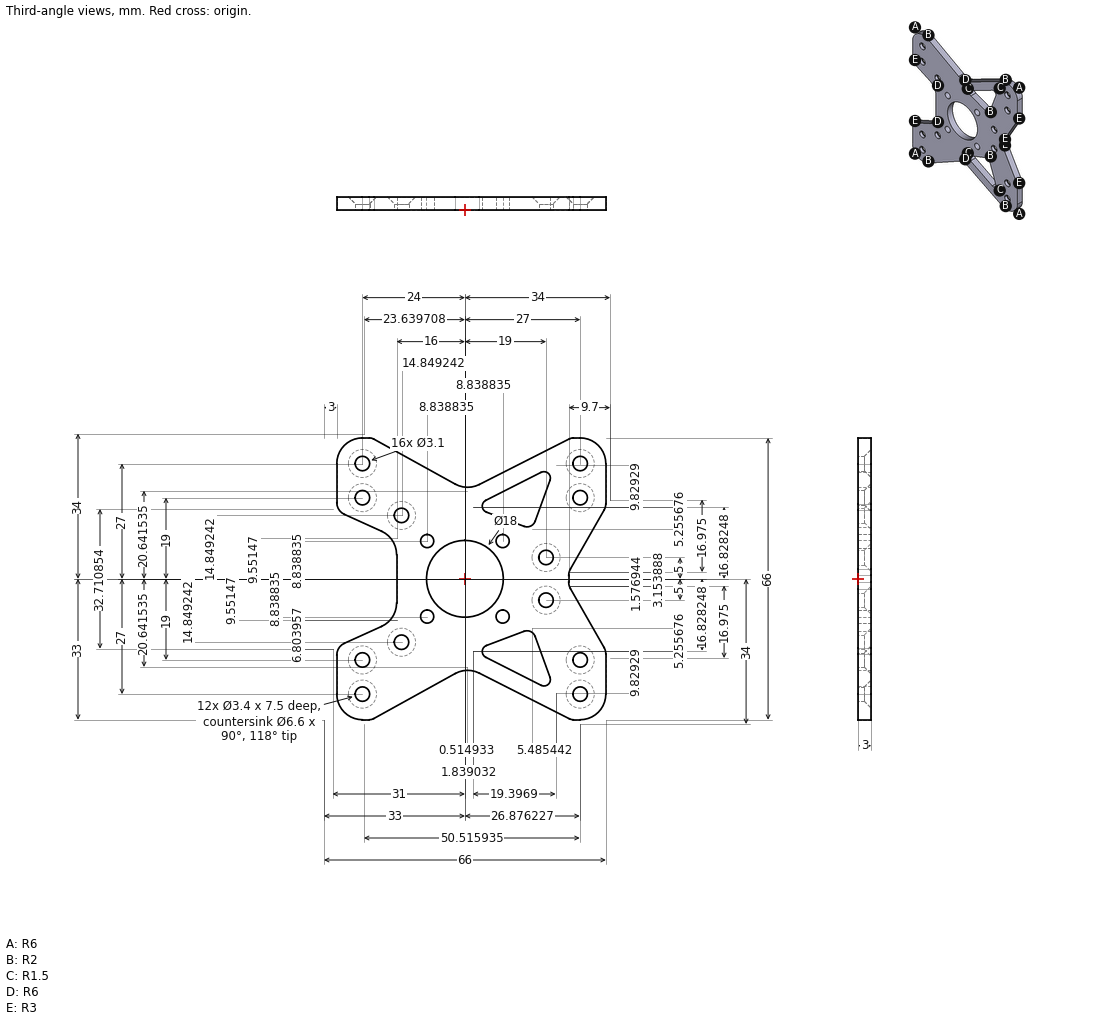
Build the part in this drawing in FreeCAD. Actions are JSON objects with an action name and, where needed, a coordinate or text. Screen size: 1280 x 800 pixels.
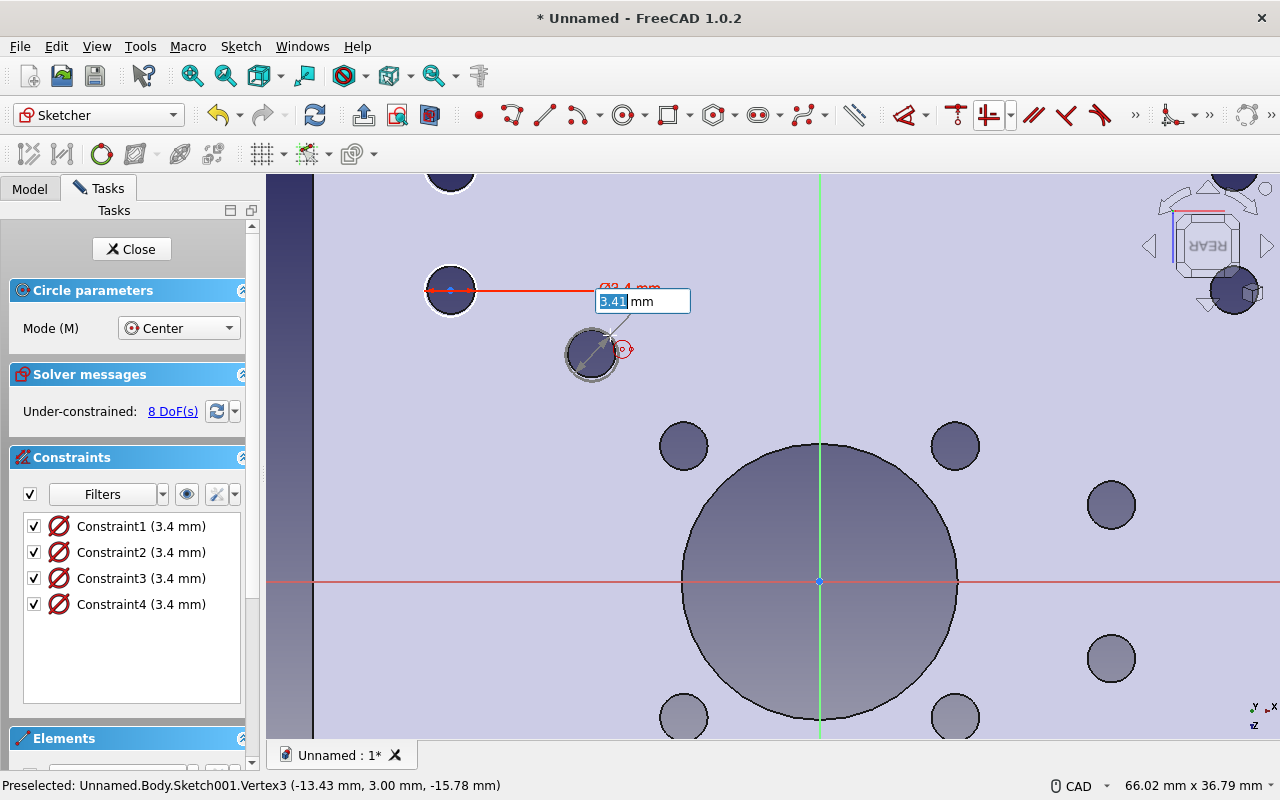
{"action": "type", "text": "3.4"}
{"action": "key", "text": "Return"}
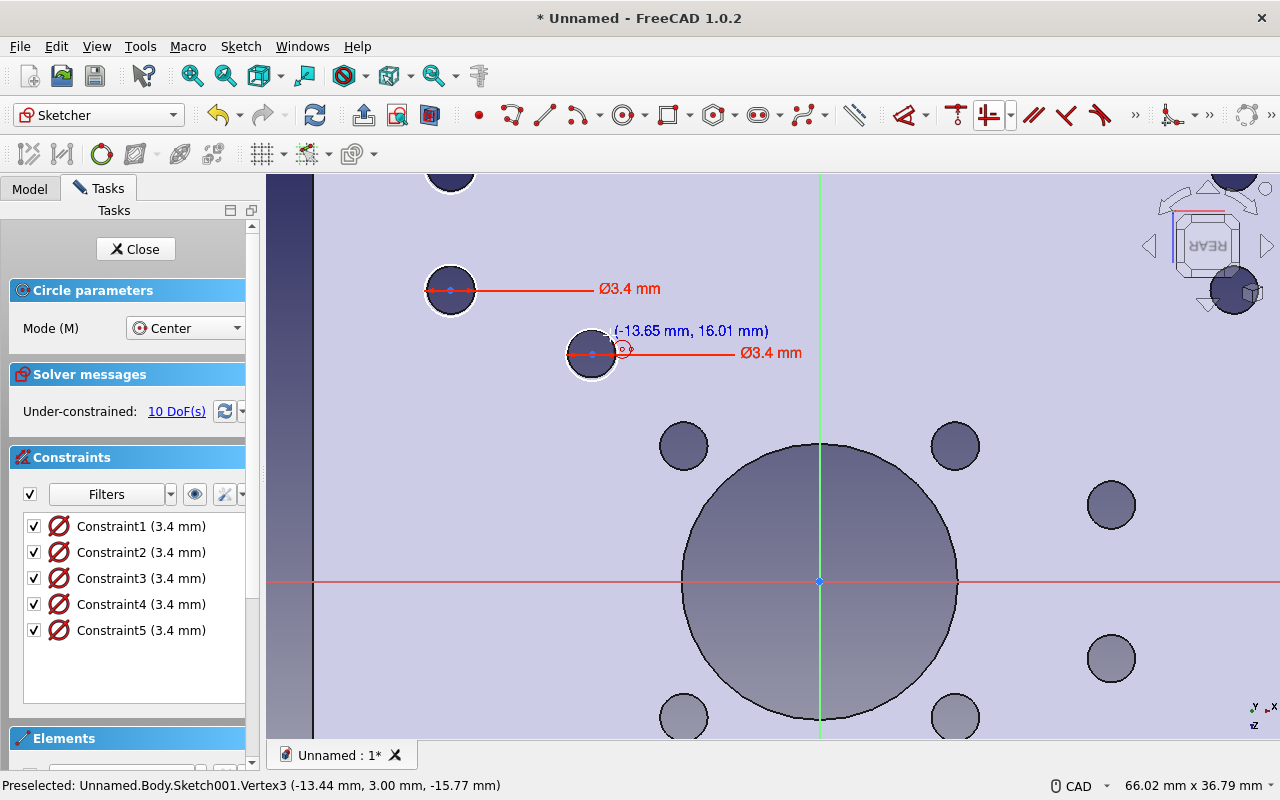
{"action": "scroll", "coordinate": [592, 354], "scroll_direction": "down", "scroll_amount": 4}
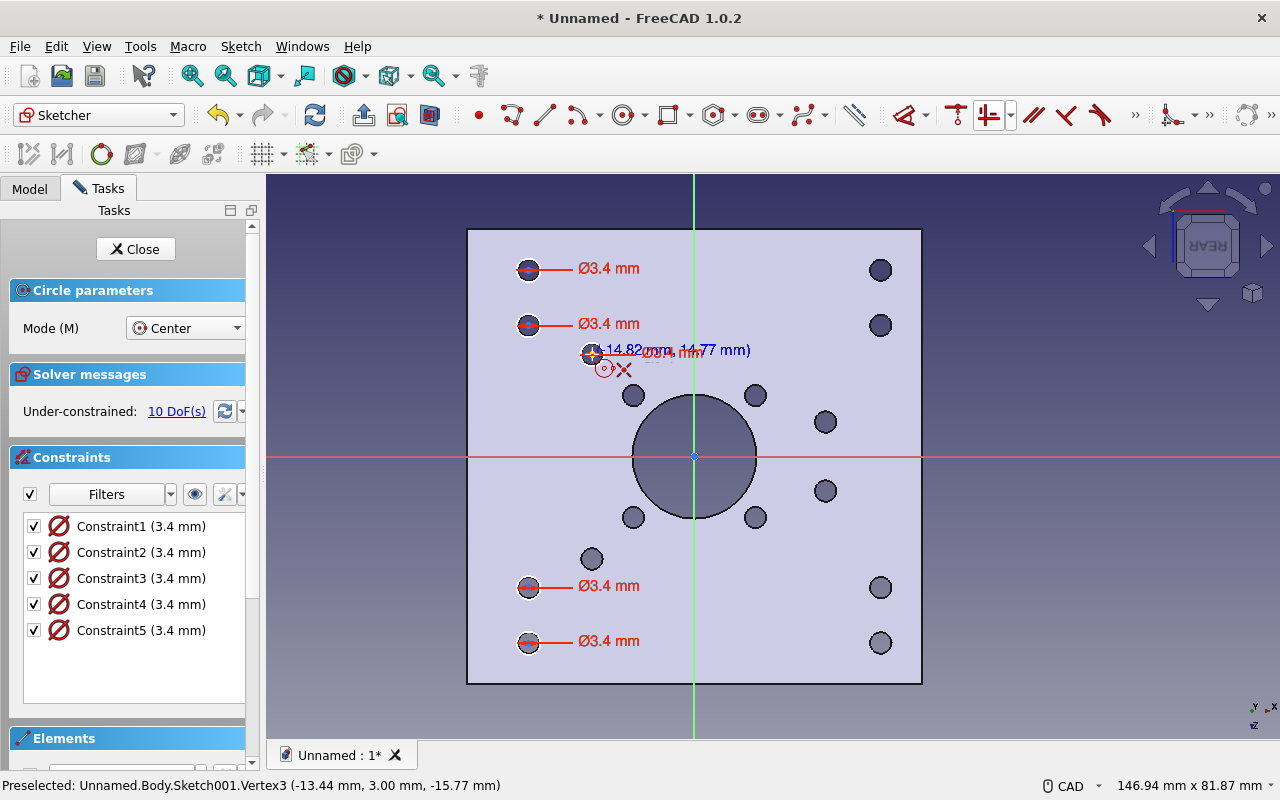
{"action": "scroll", "coordinate": [592, 559], "scroll_direction": "up", "scroll_amount": 4}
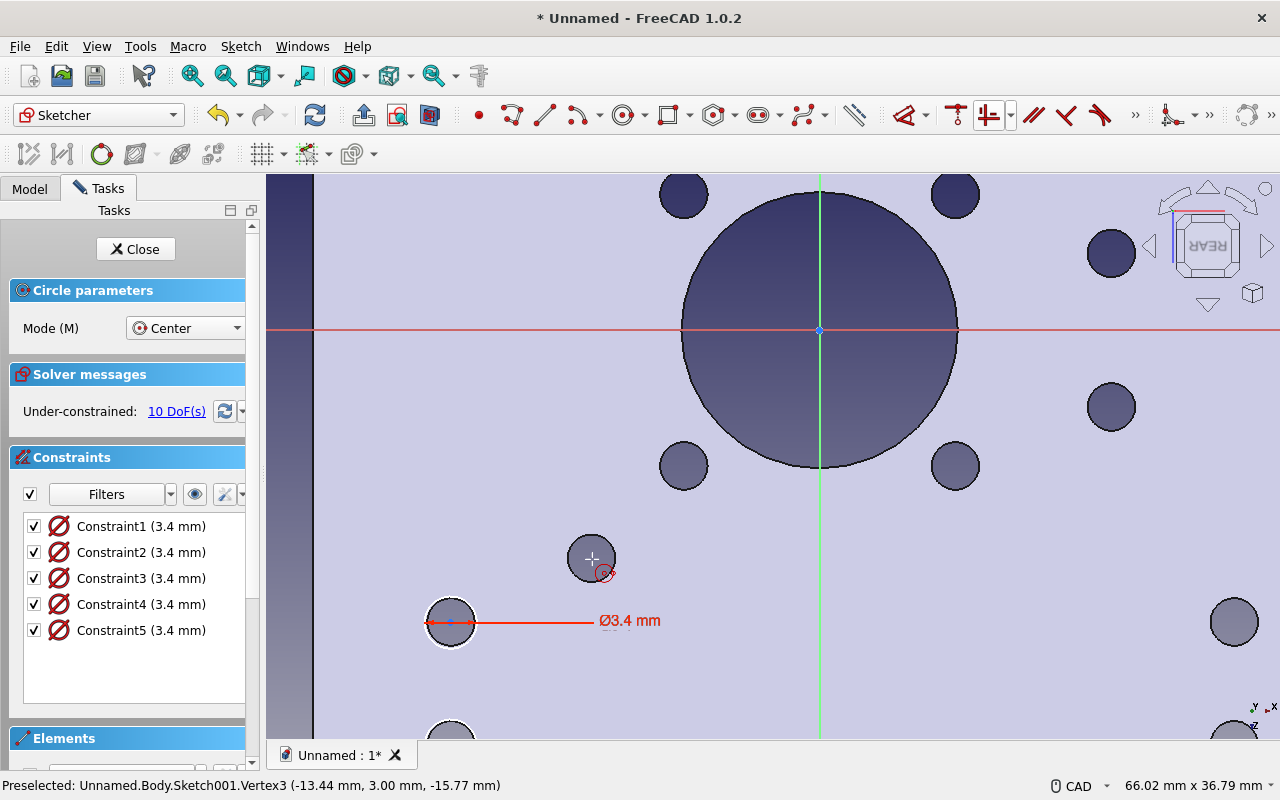
{"action": "left_click", "coordinate": [592, 558]}
{"action": "mouse_move", "coordinate": [610, 540]}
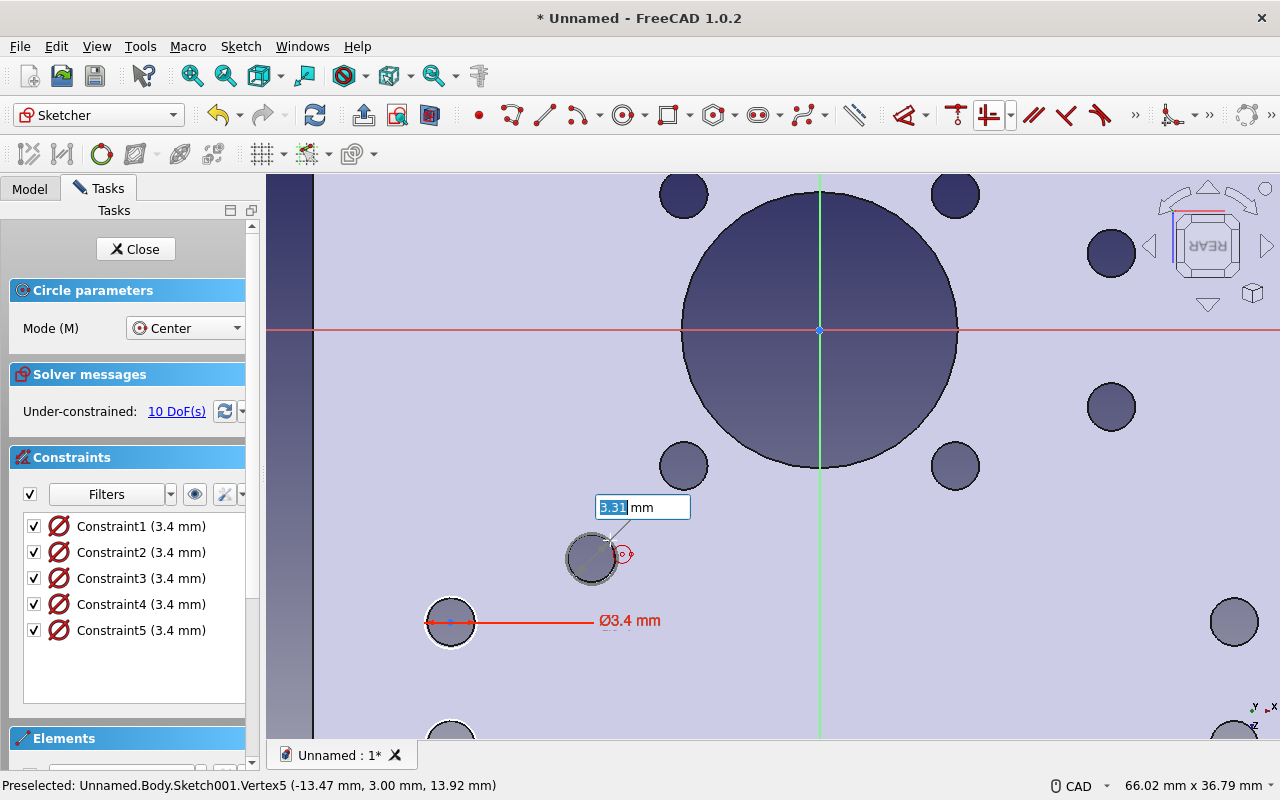
{"action": "type", "text": "3.4"}
{"action": "key", "text": "Return"}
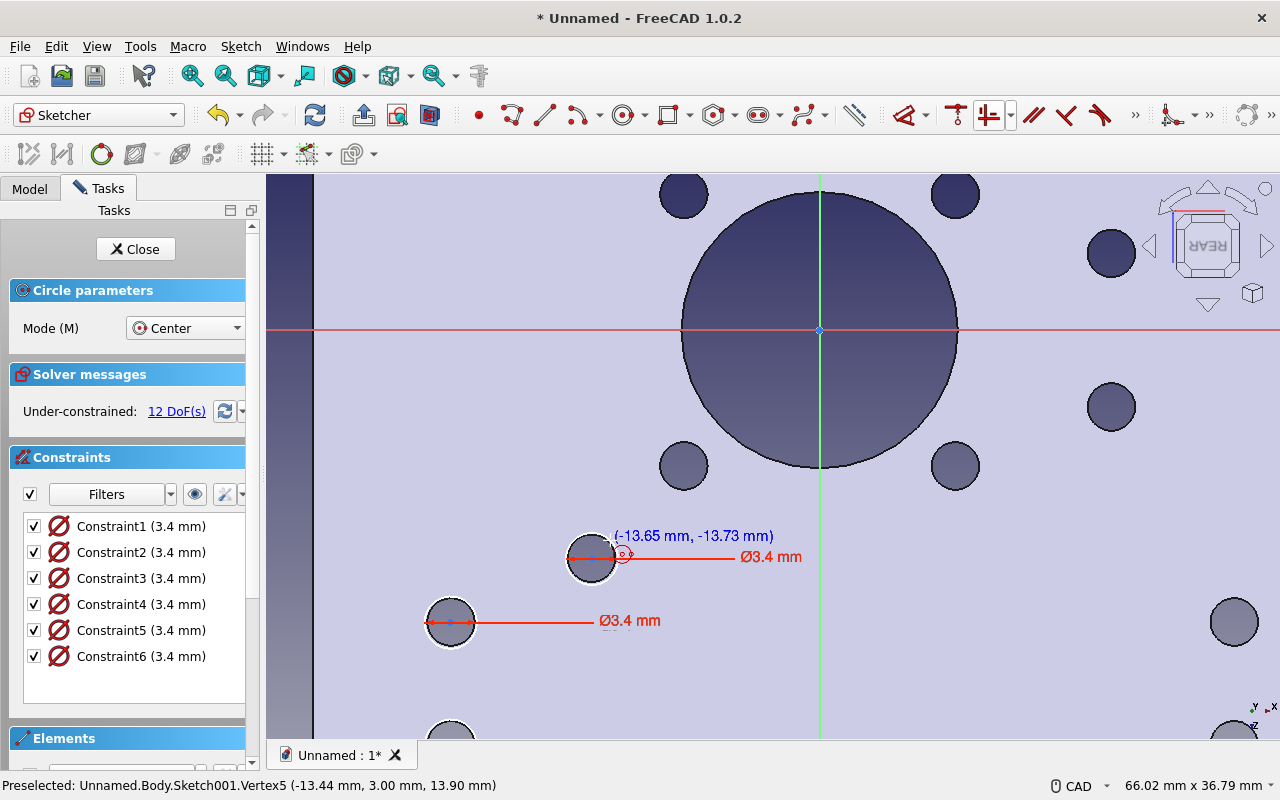
{"action": "left_click", "coordinate": [1111, 407]}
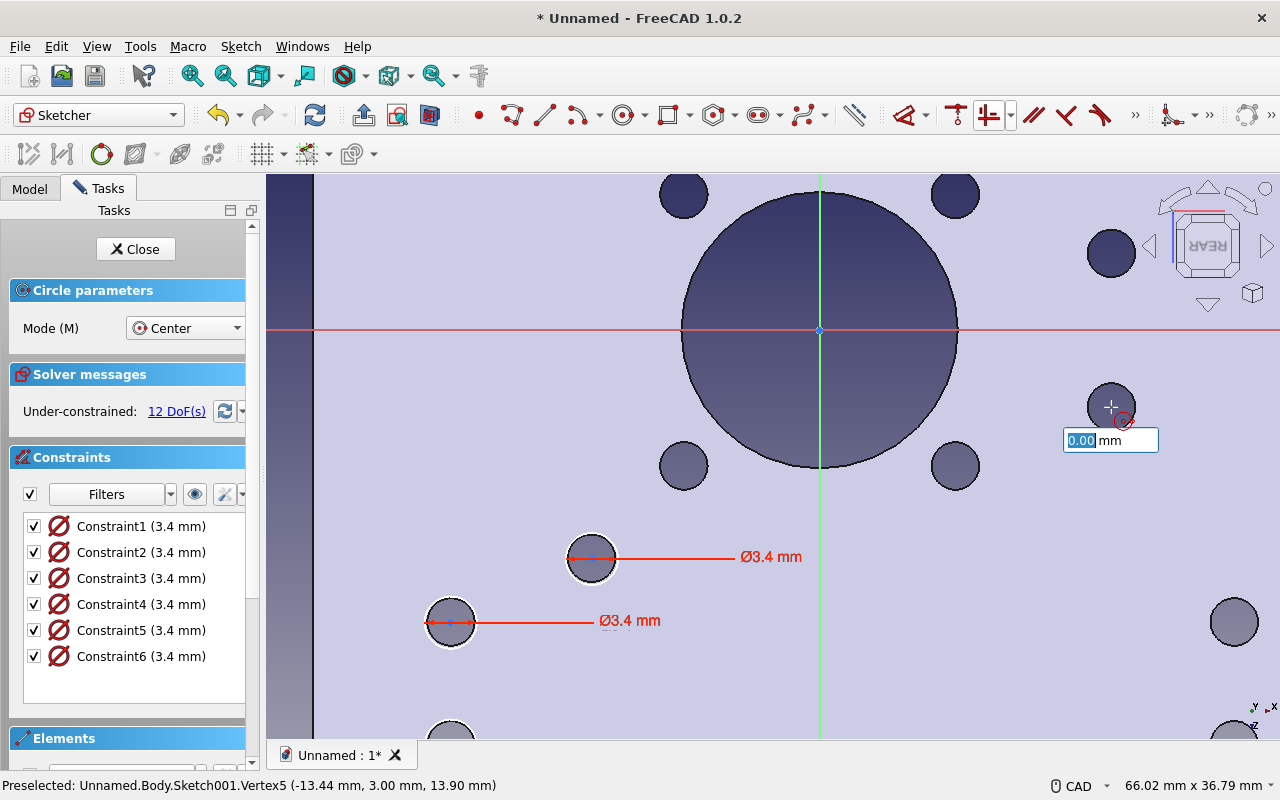
{"action": "scroll", "coordinate": [592, 560], "scroll_direction": "down", "scroll_amount": 4}
{"action": "mouse_move", "coordinate": [834, 483]}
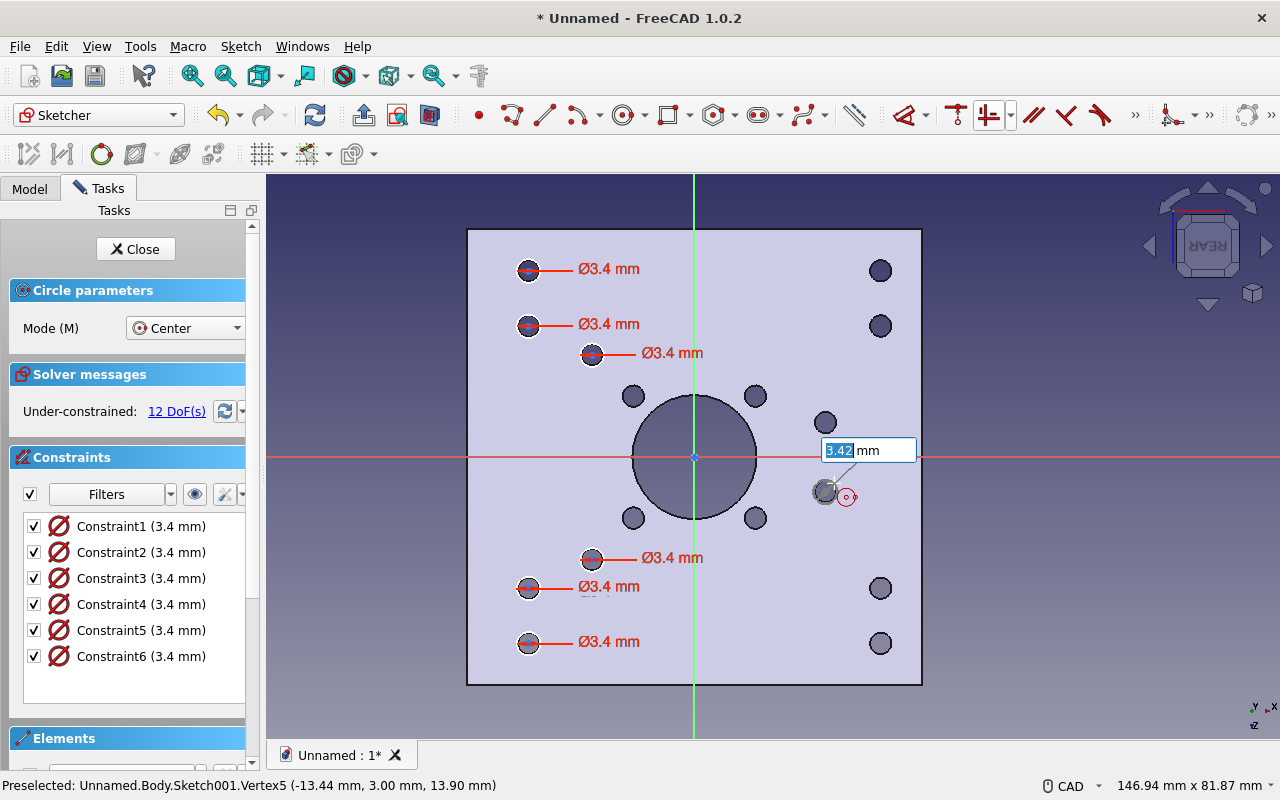
{"action": "type", "text": "3.4"}
{"action": "key", "text": "Return"}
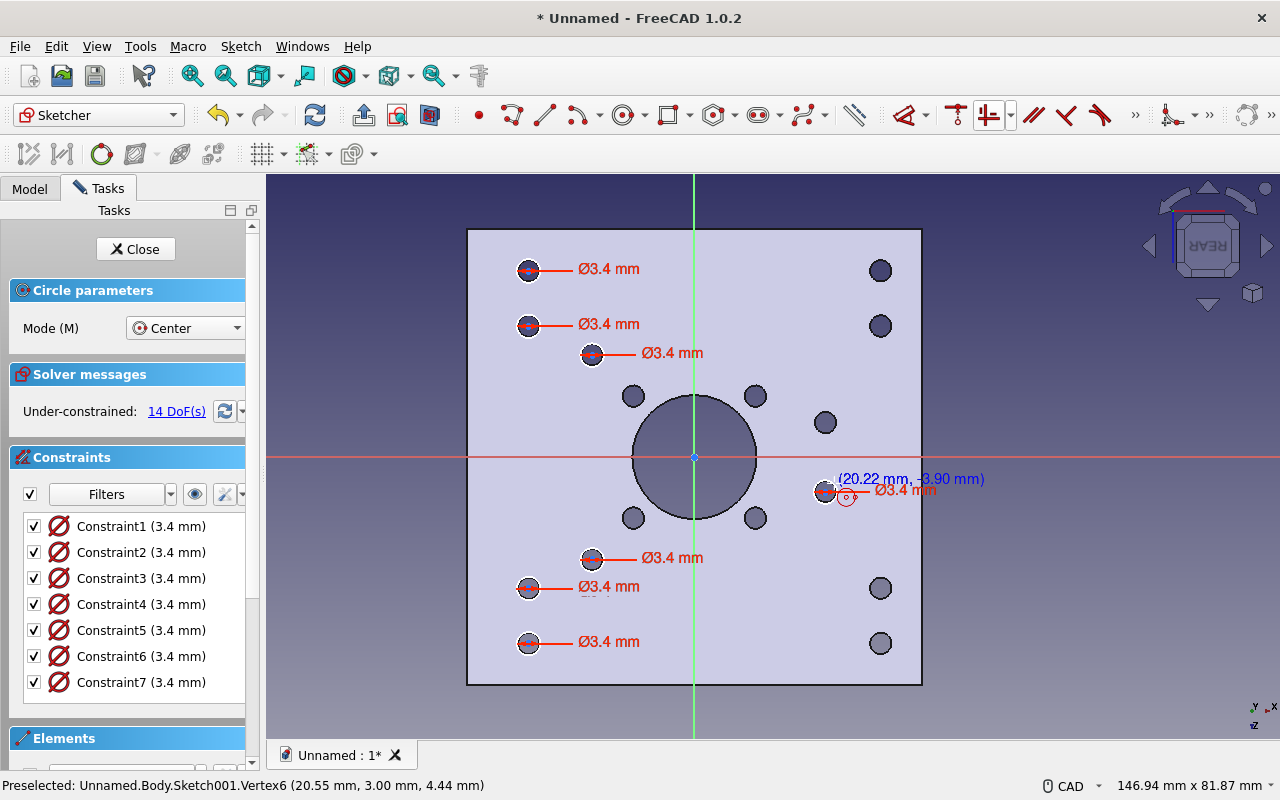
{"action": "scroll", "coordinate": [826, 423], "scroll_direction": "up", "scroll_amount": 4}